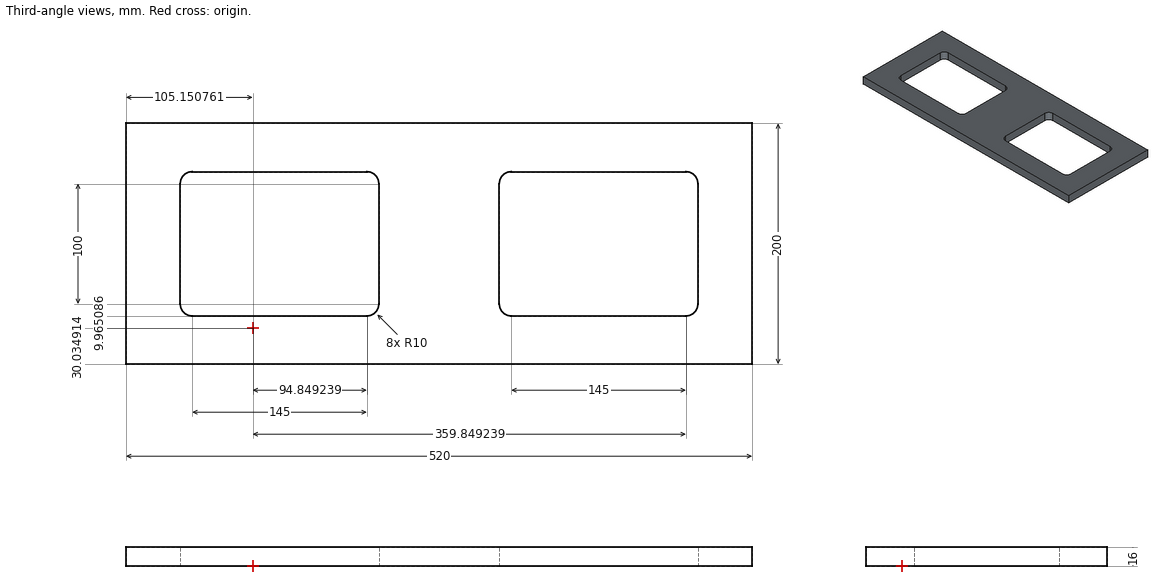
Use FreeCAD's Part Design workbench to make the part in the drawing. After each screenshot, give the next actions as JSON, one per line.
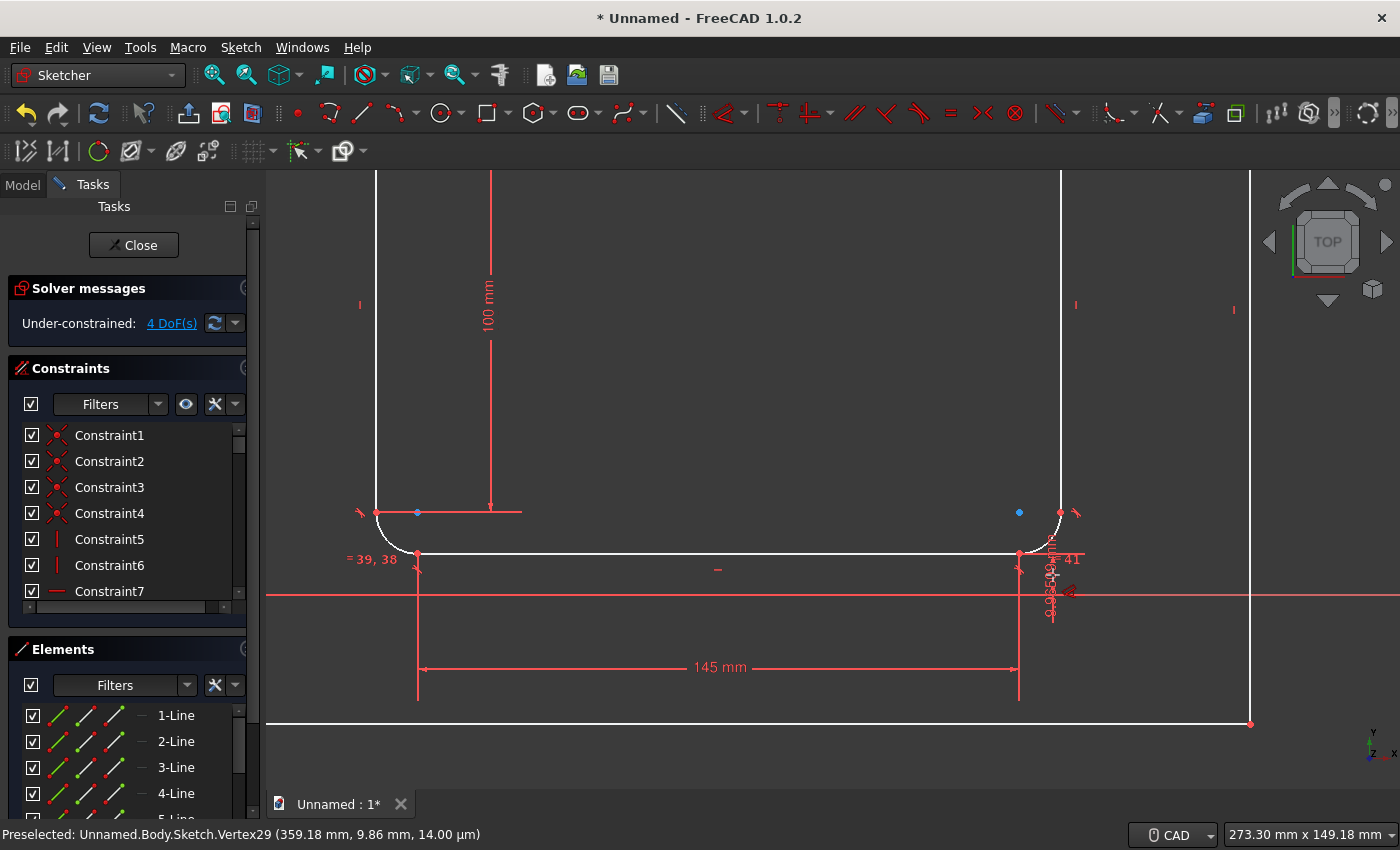
{"action": "scroll", "coordinate": [1020, 555], "scroll_direction": "down", "scroll_amount": 6}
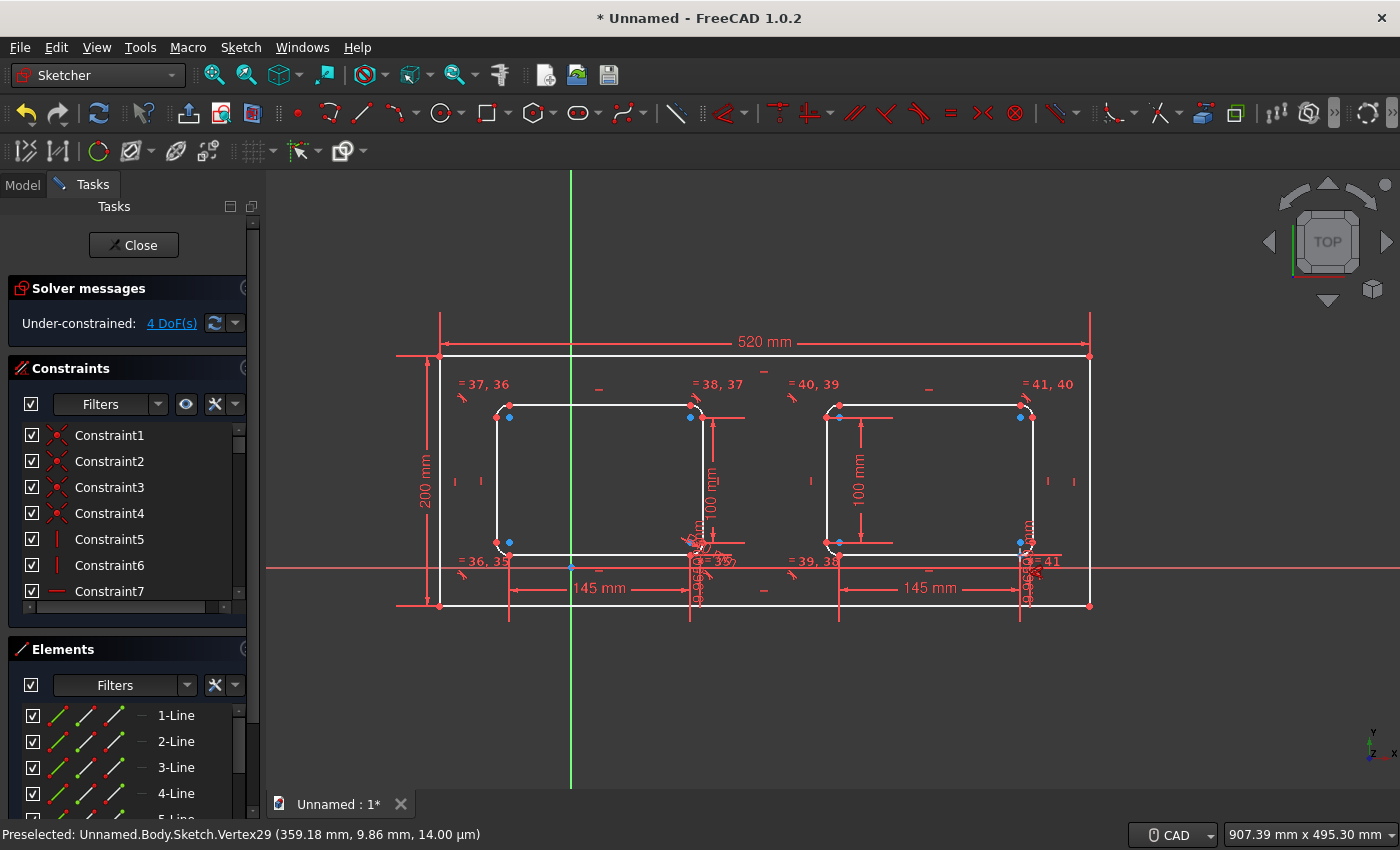
{"action": "left_click", "coordinate": [440, 606]}
{"action": "left_click", "coordinate": [406, 587]}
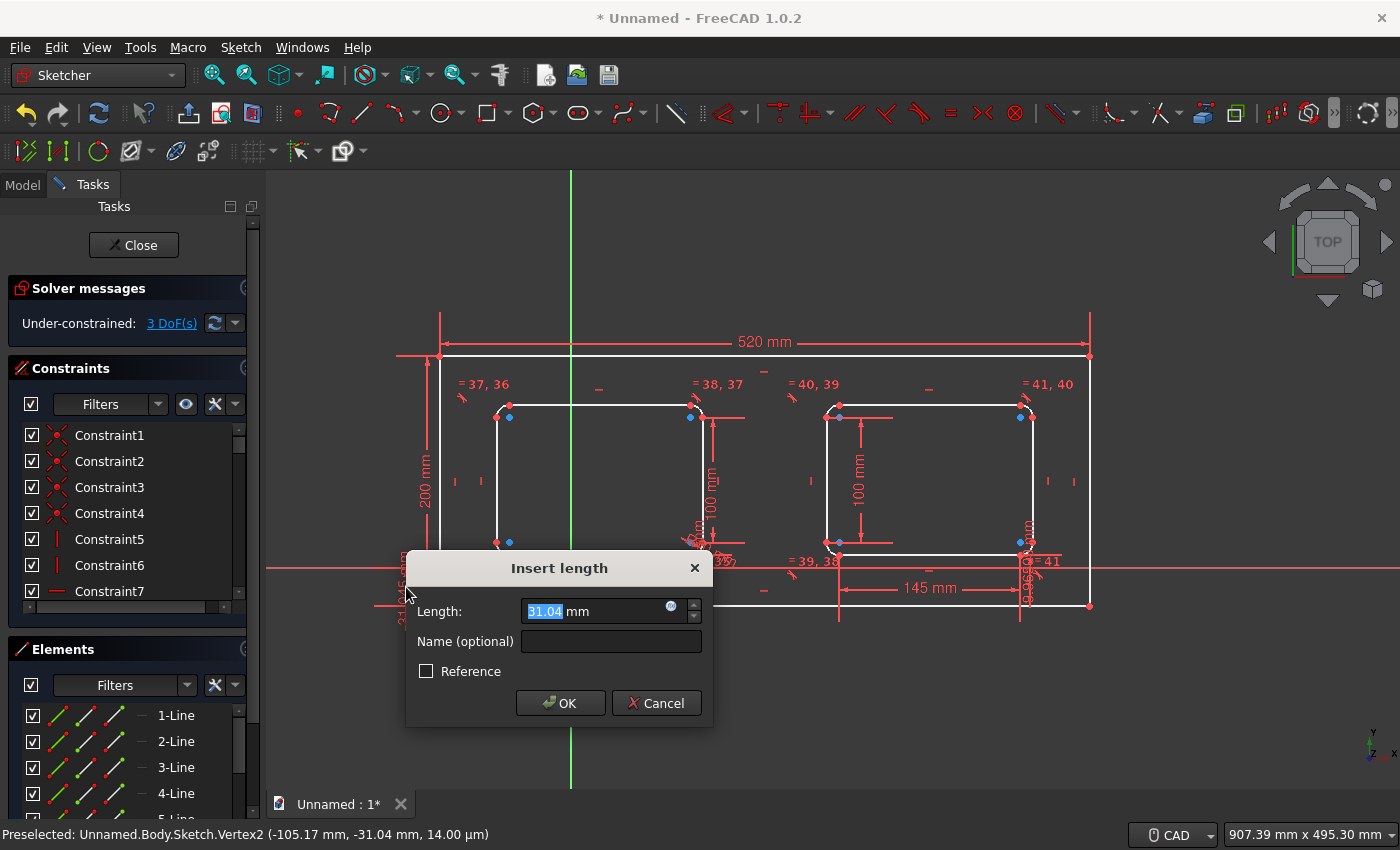
{"action": "type", "text": "30.034914"}
{"action": "key", "text": "Return"}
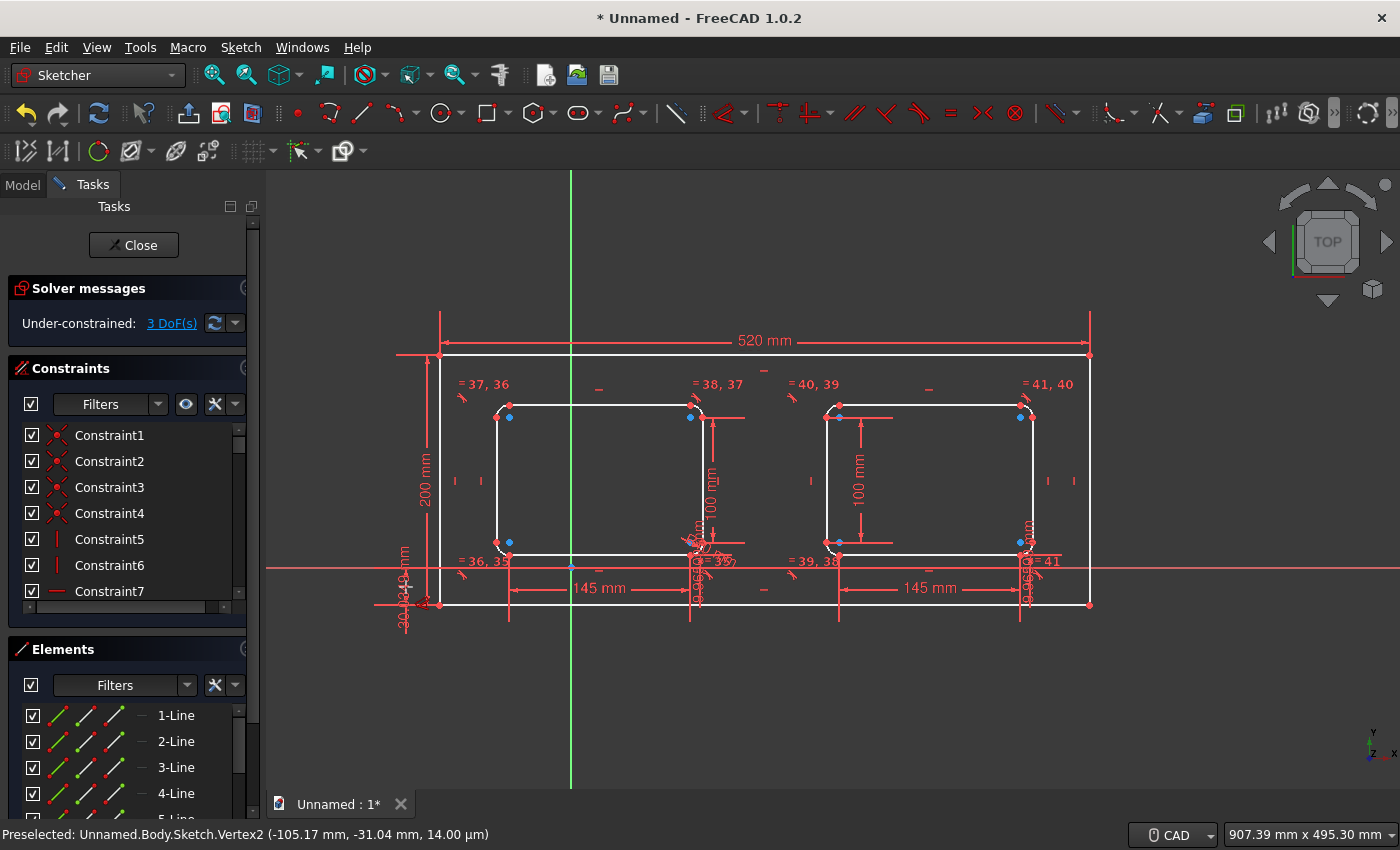
{"action": "left_click", "coordinate": [690, 555]}
{"action": "left_click", "coordinate": [631, 521]}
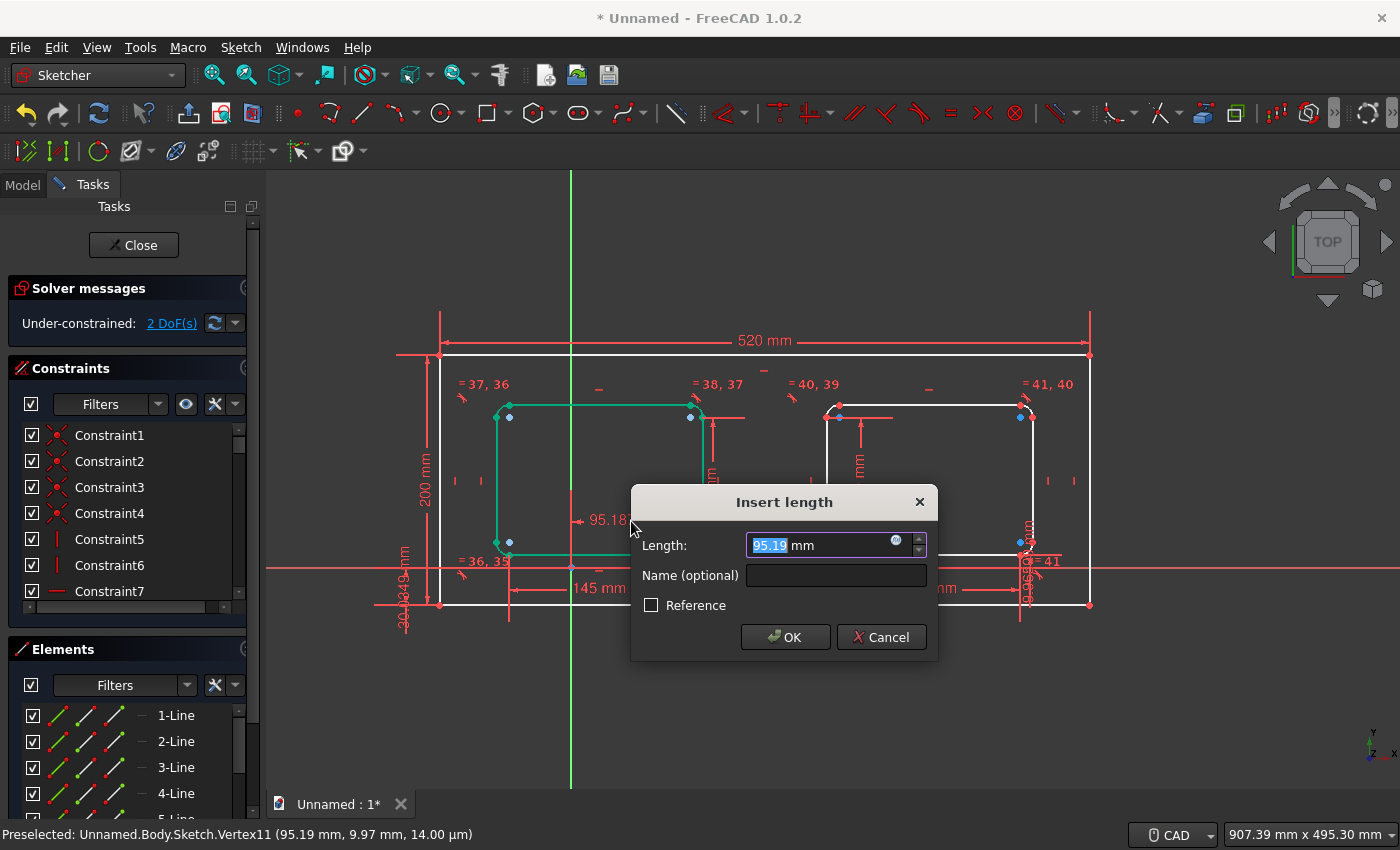
{"action": "type", "text": "94.849239"}
{"action": "key", "text": "Return"}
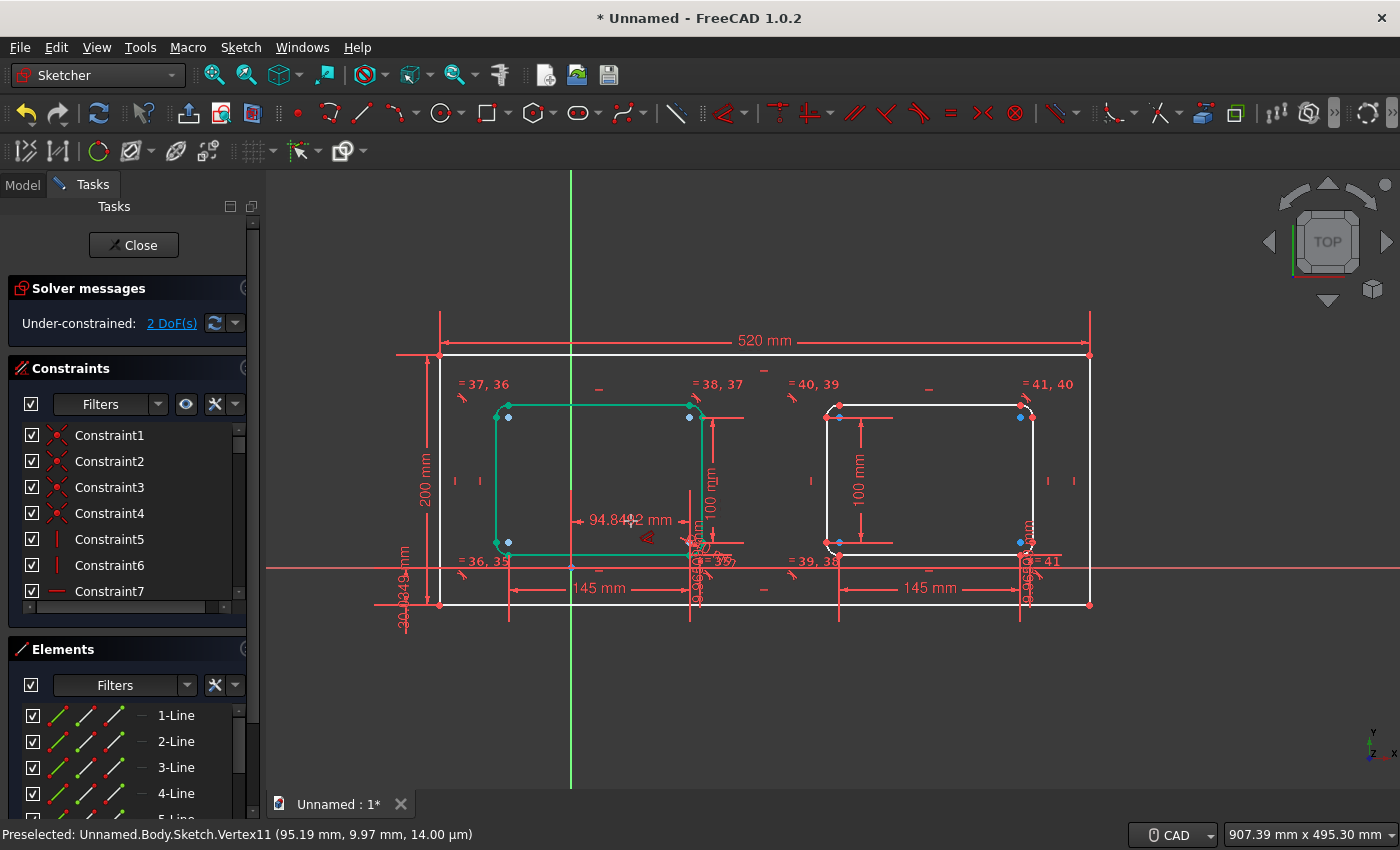
{"action": "left_click", "coordinate": [440, 355]}
{"action": "left_click", "coordinate": [506, 321]}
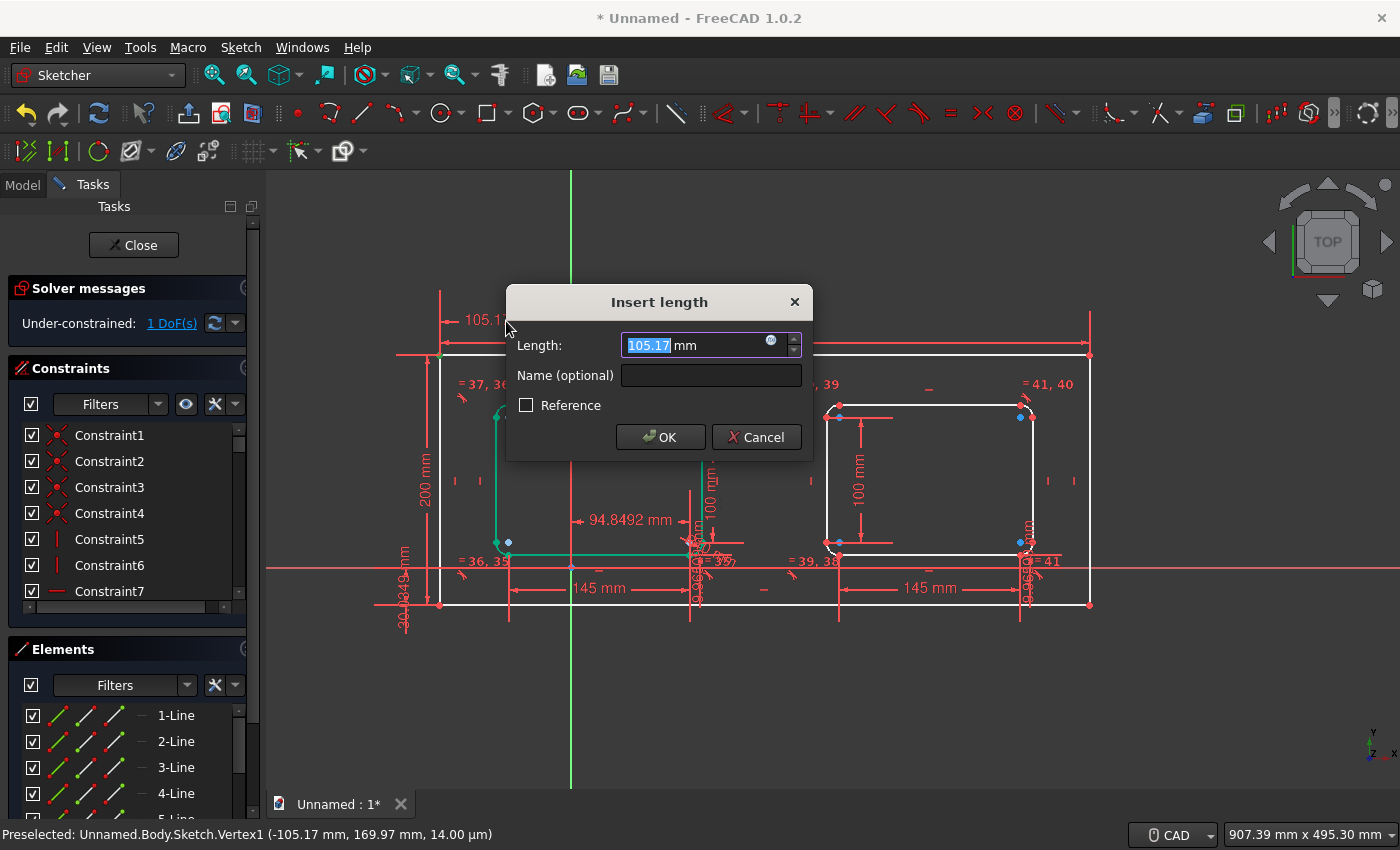
{"action": "type", "text": "105.150761"}
{"action": "key", "text": "Return"}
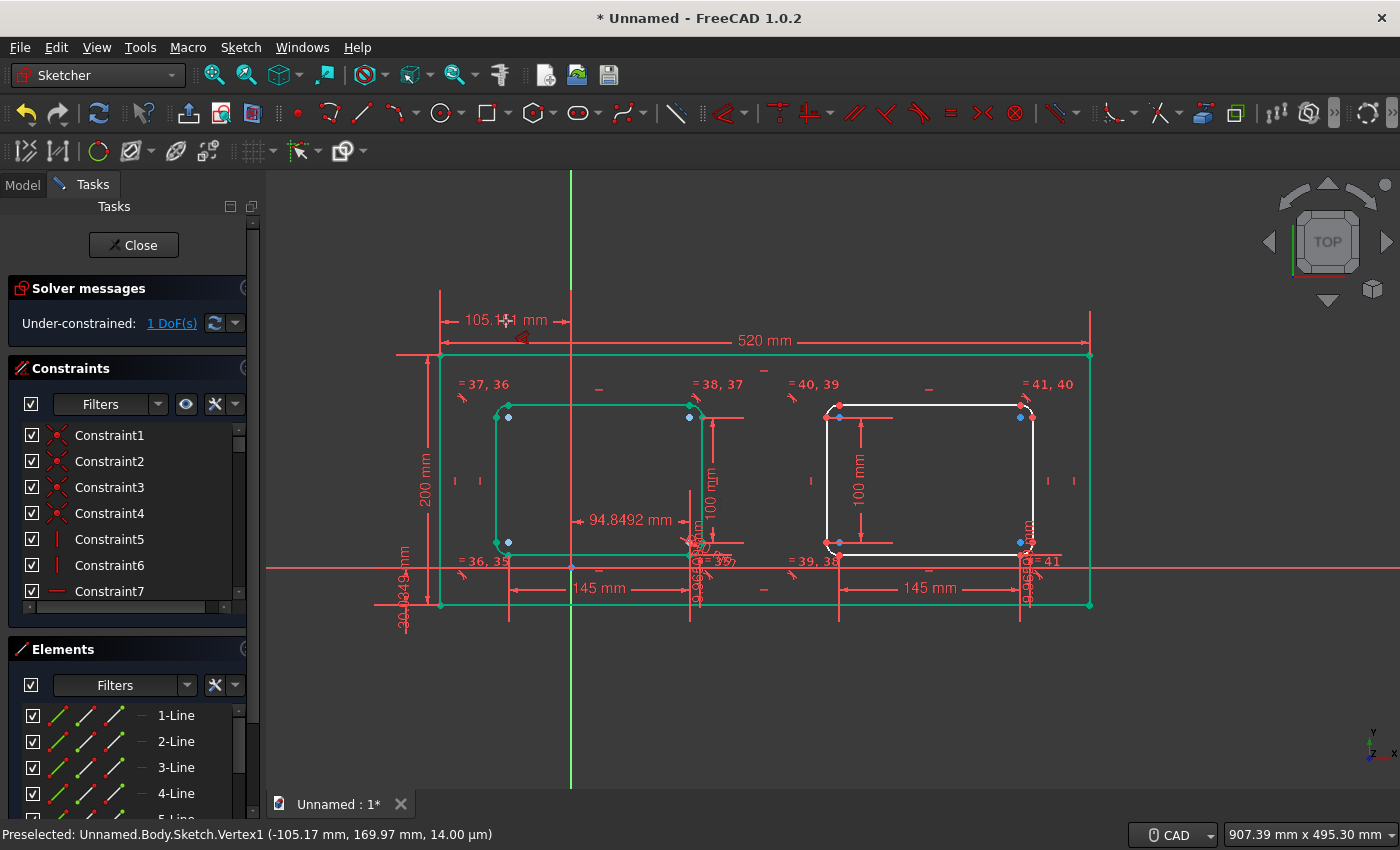
{"action": "left_click", "coordinate": [1020, 555]}
{"action": "left_click", "coordinate": [796, 521]}